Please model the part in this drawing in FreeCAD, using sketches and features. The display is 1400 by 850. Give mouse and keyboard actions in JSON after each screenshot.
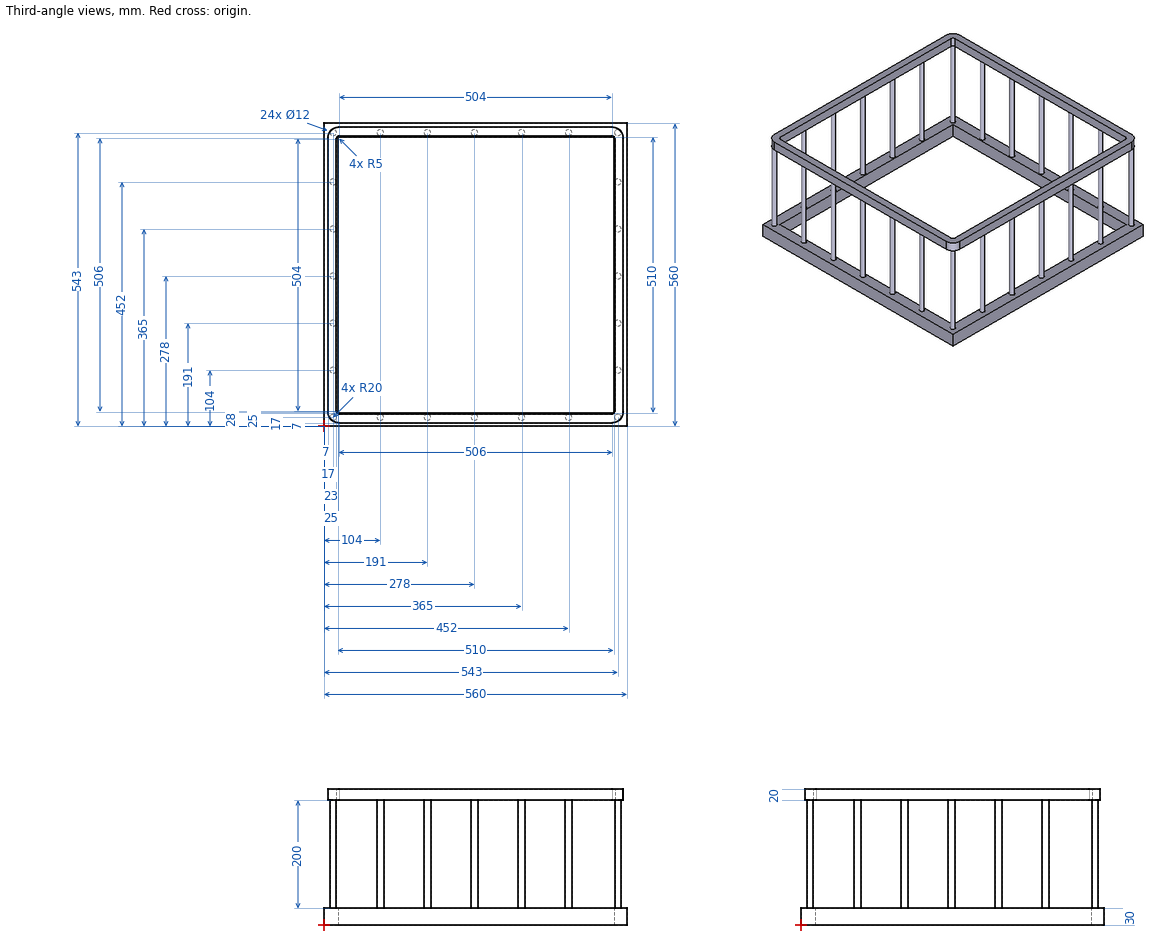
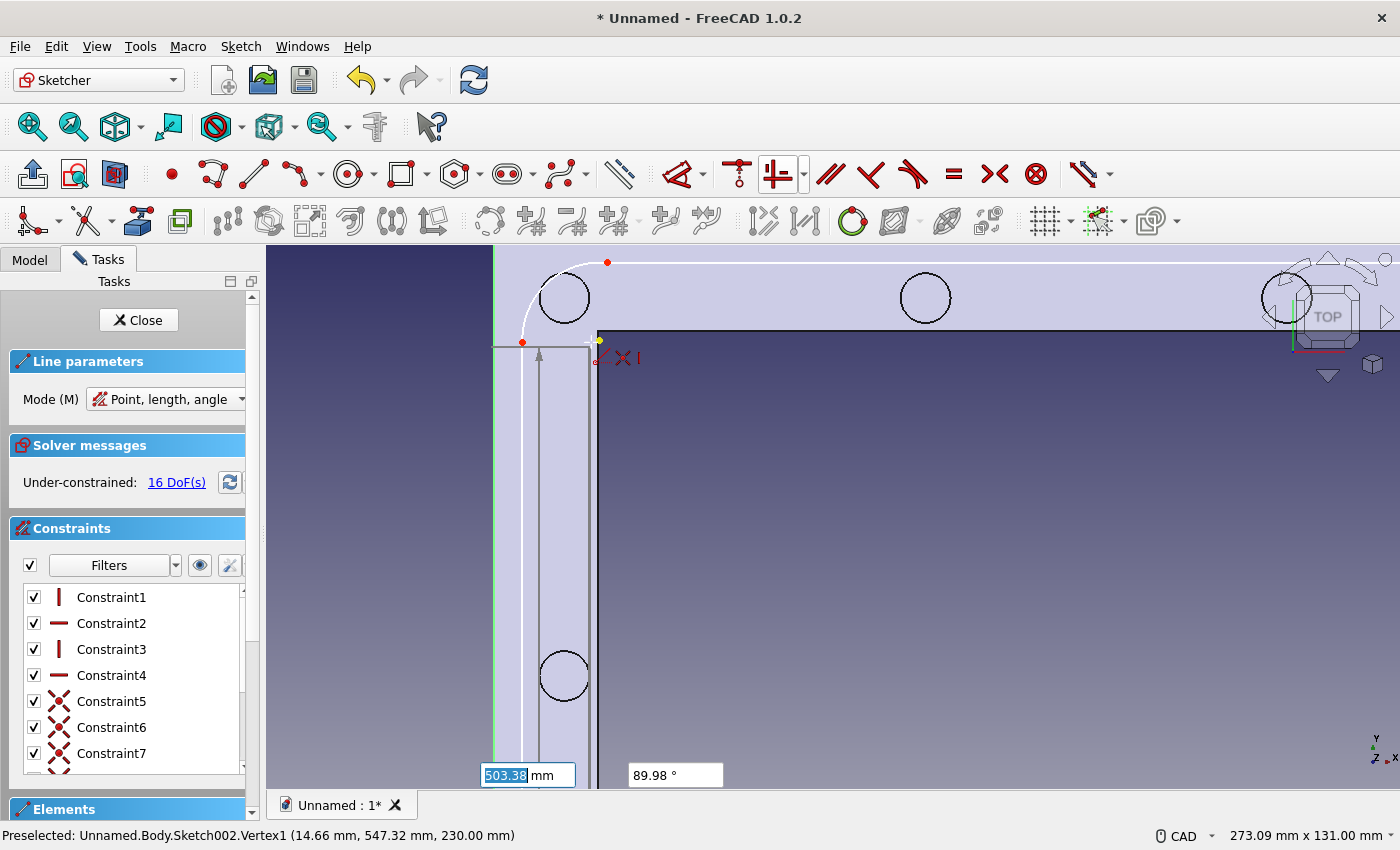
{"action": "left_click", "coordinate": [589, 344]}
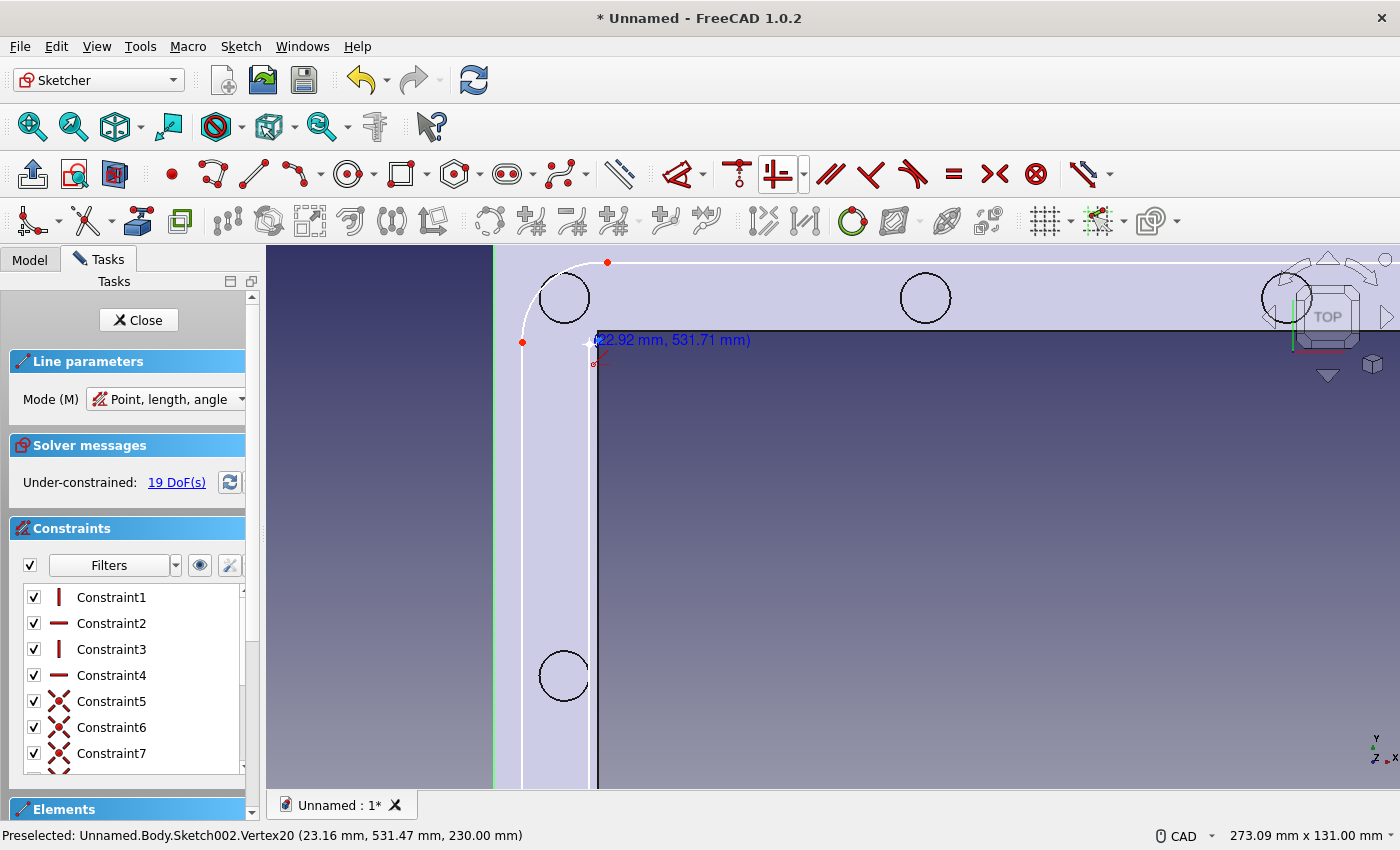
{"action": "left_click", "coordinate": [610, 323]}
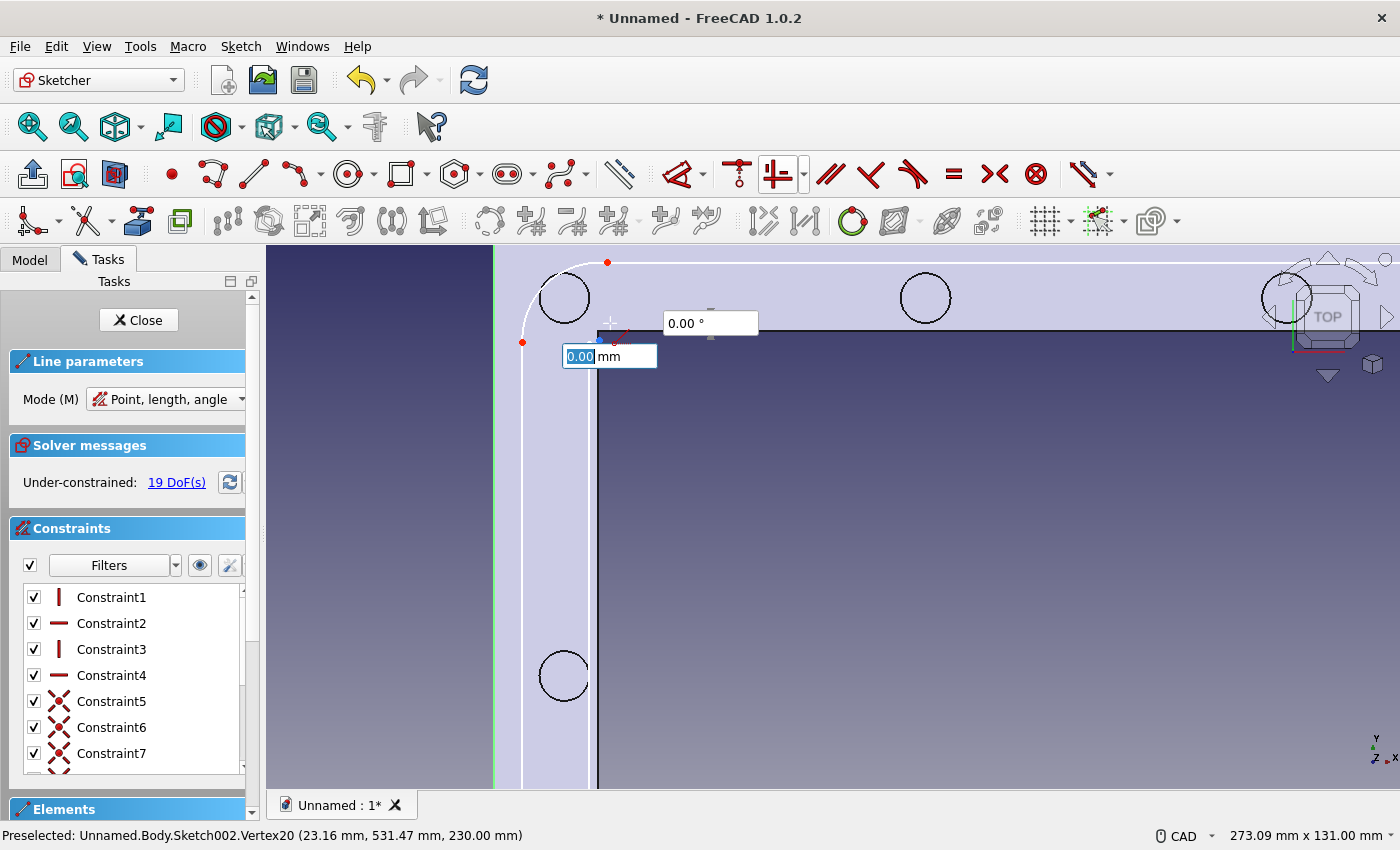
{"action": "scroll", "coordinate": [591, 341], "scroll_direction": "down", "scroll_amount": 9}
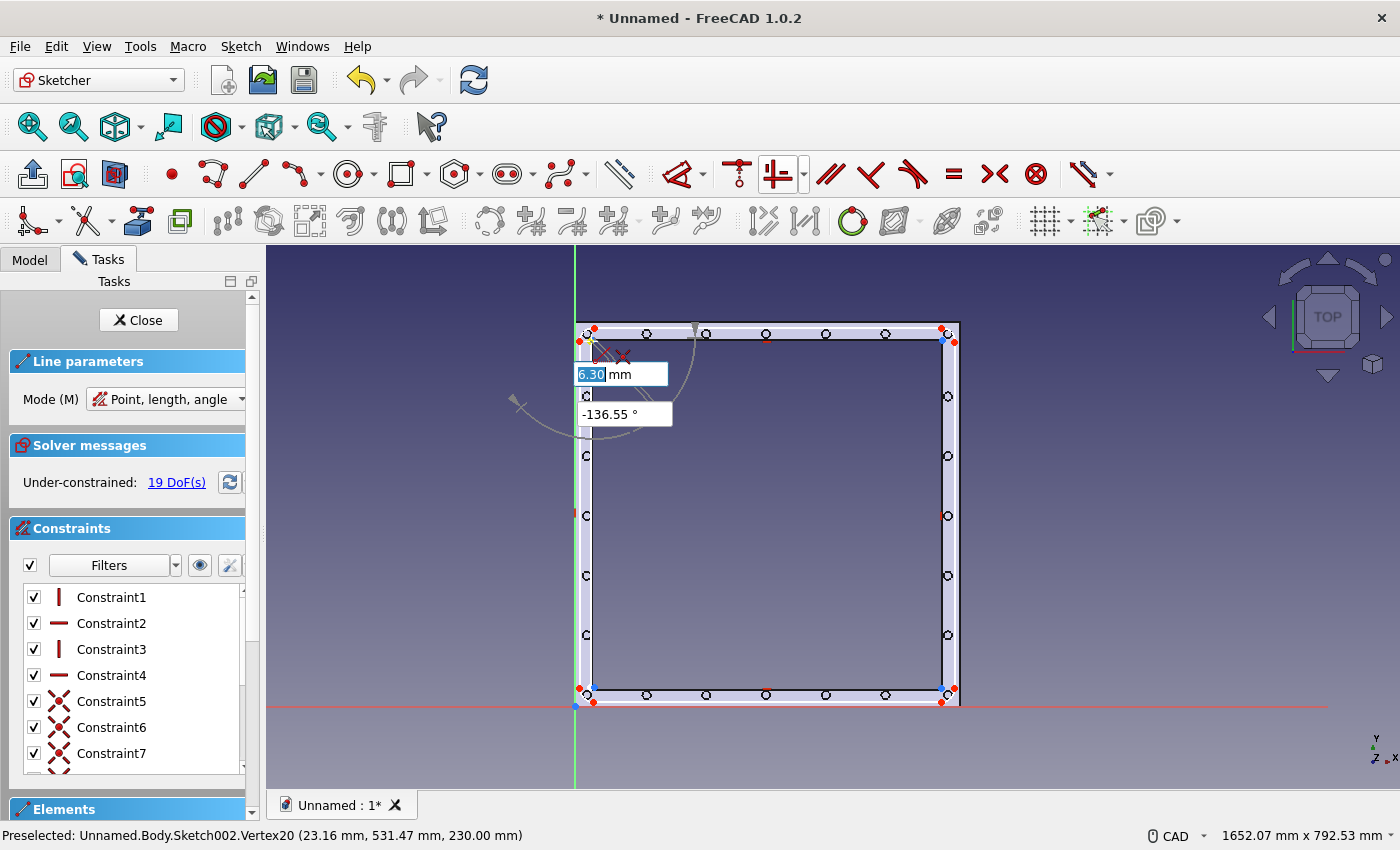
{"action": "scroll", "coordinate": [940, 338], "scroll_direction": "up", "scroll_amount": 9}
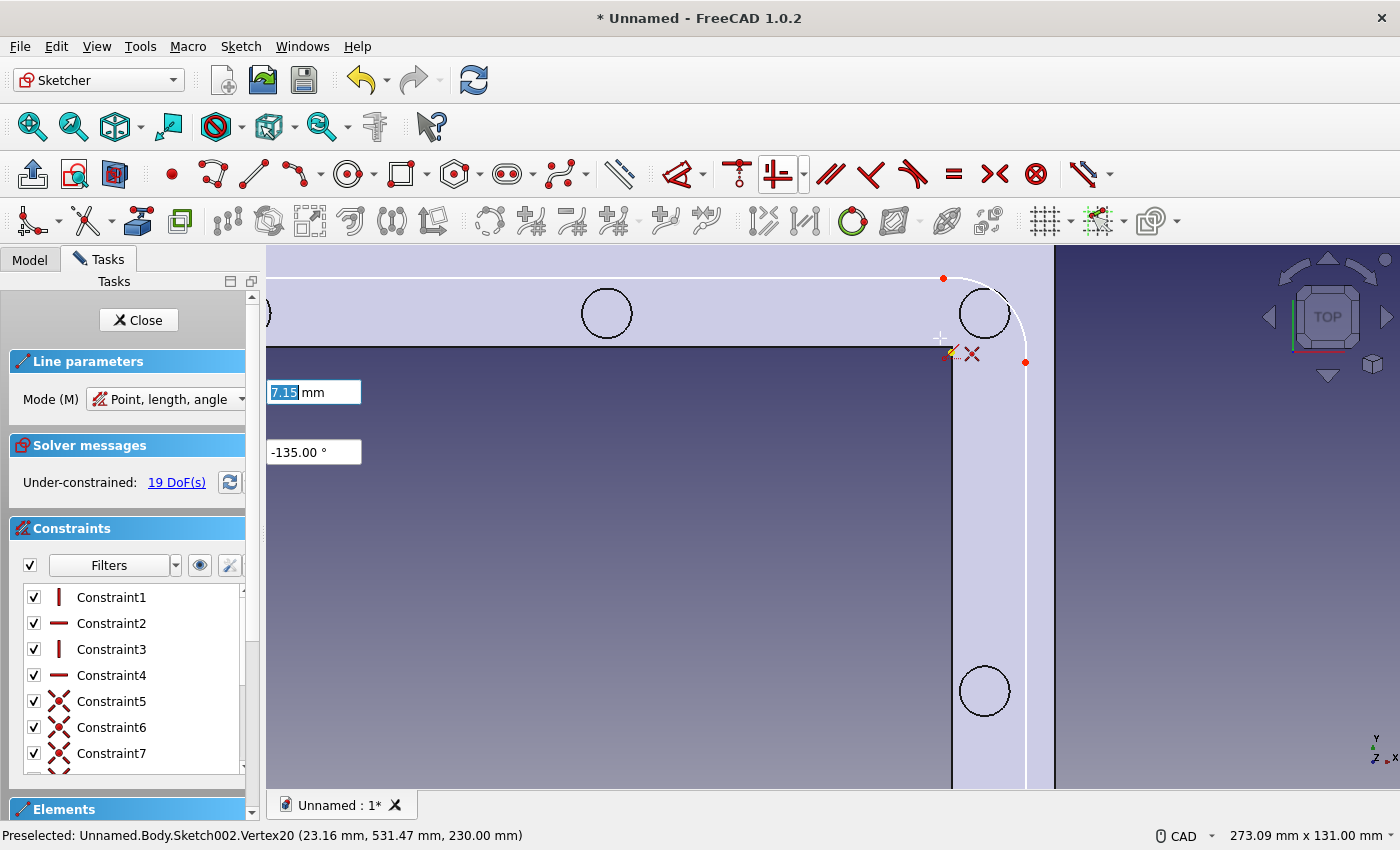
{"action": "left_click", "coordinate": [939, 338]}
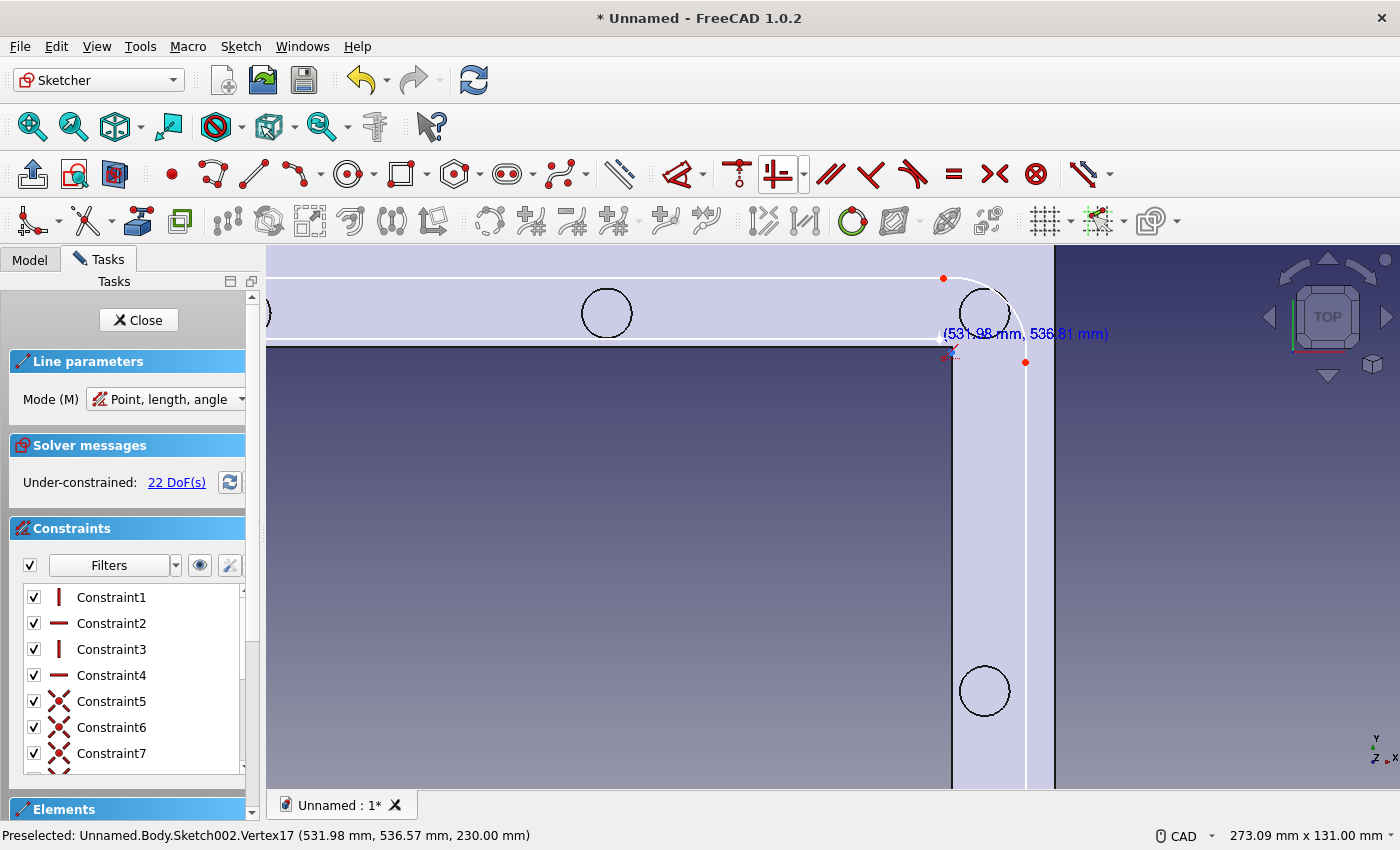
{"action": "left_click", "coordinate": [960, 359]}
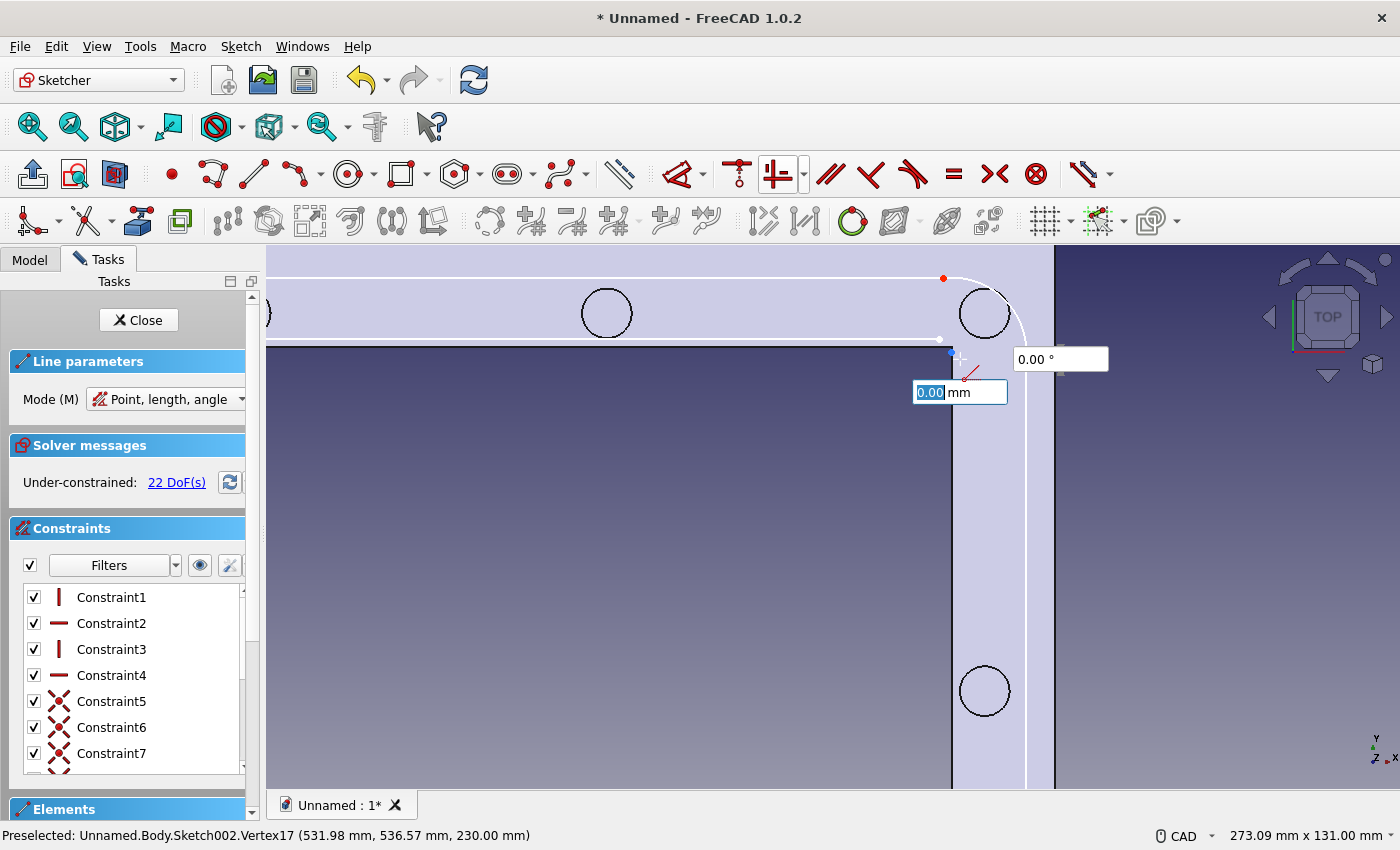
{"action": "scroll", "coordinate": [940, 338], "scroll_direction": "down", "scroll_amount": 9}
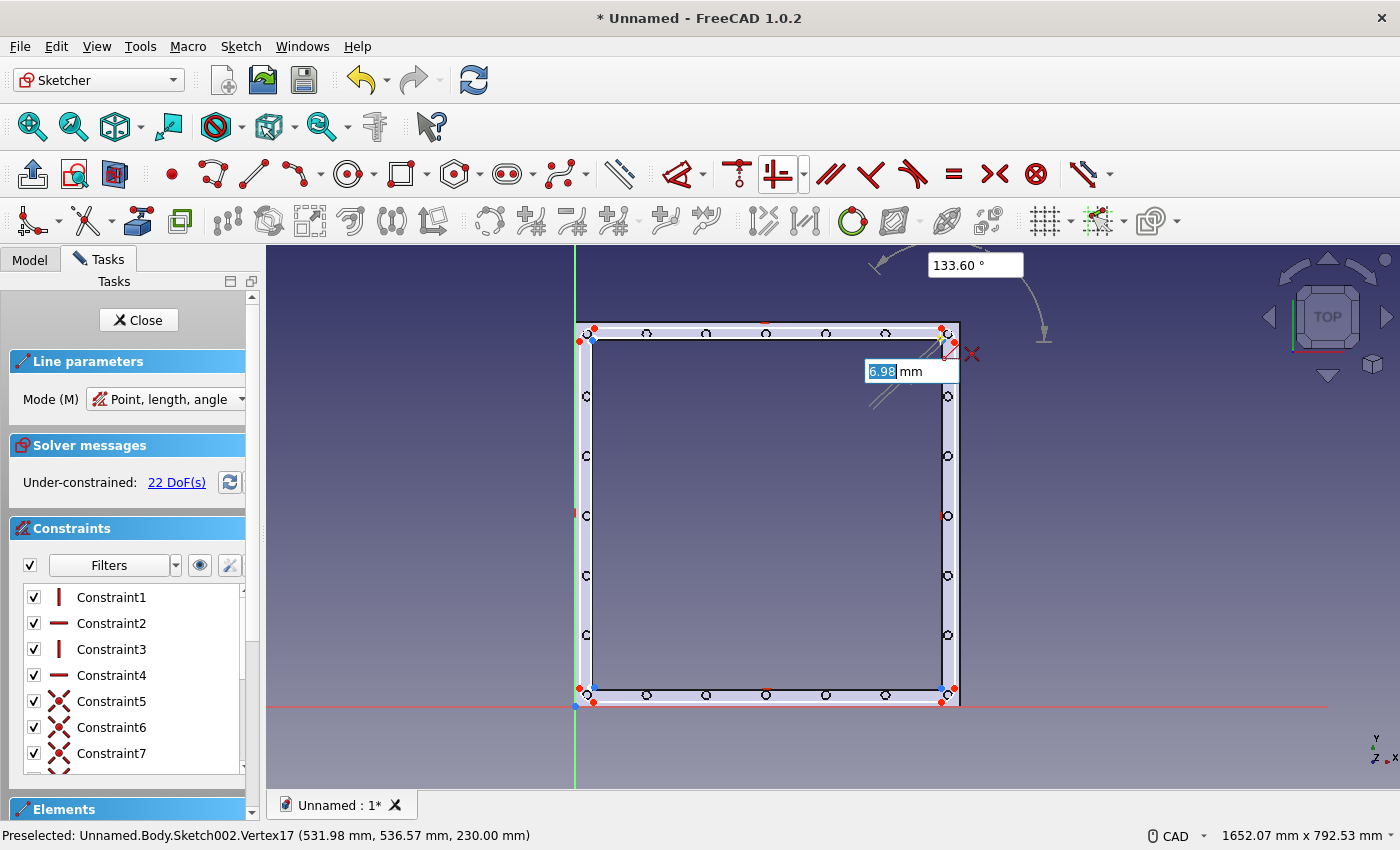
{"action": "scroll", "coordinate": [944, 688], "scroll_direction": "up", "scroll_amount": 9}